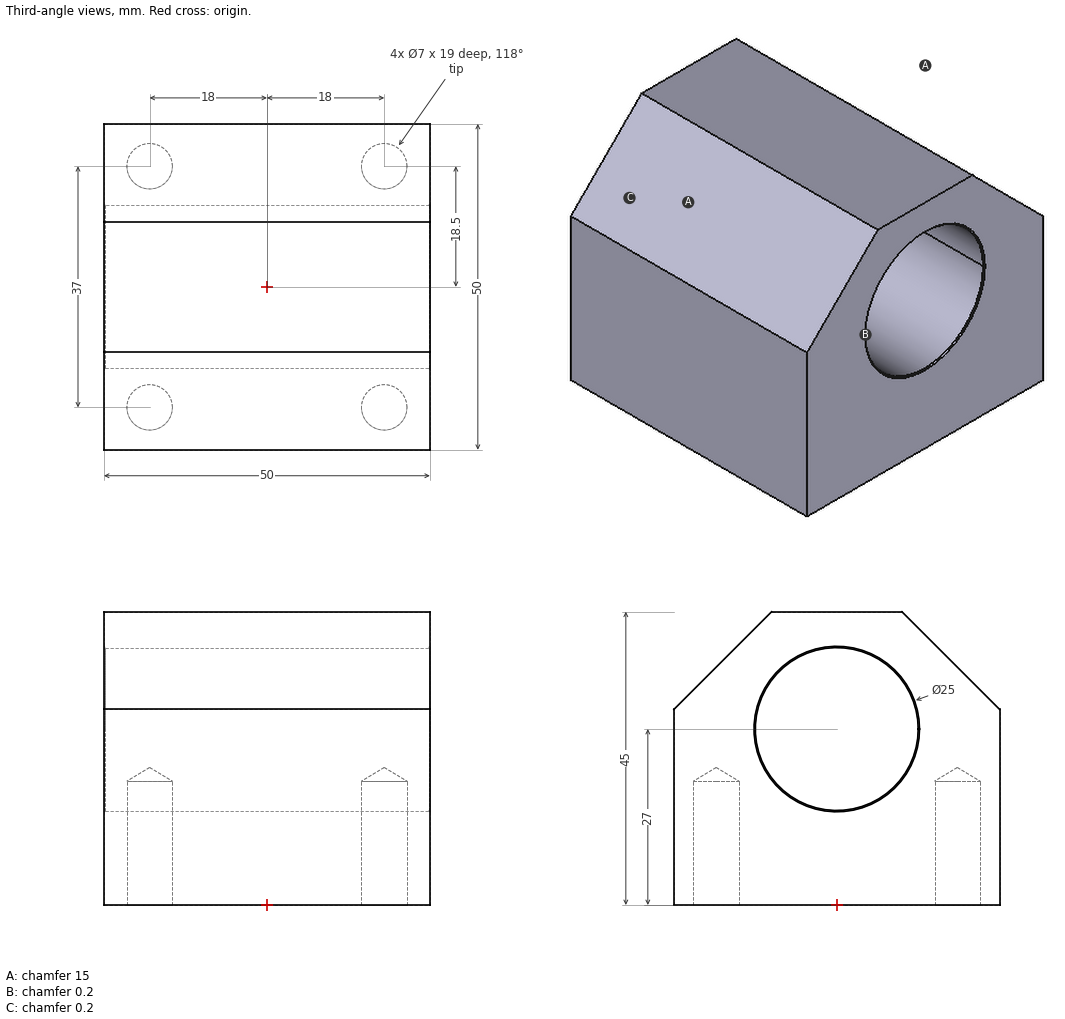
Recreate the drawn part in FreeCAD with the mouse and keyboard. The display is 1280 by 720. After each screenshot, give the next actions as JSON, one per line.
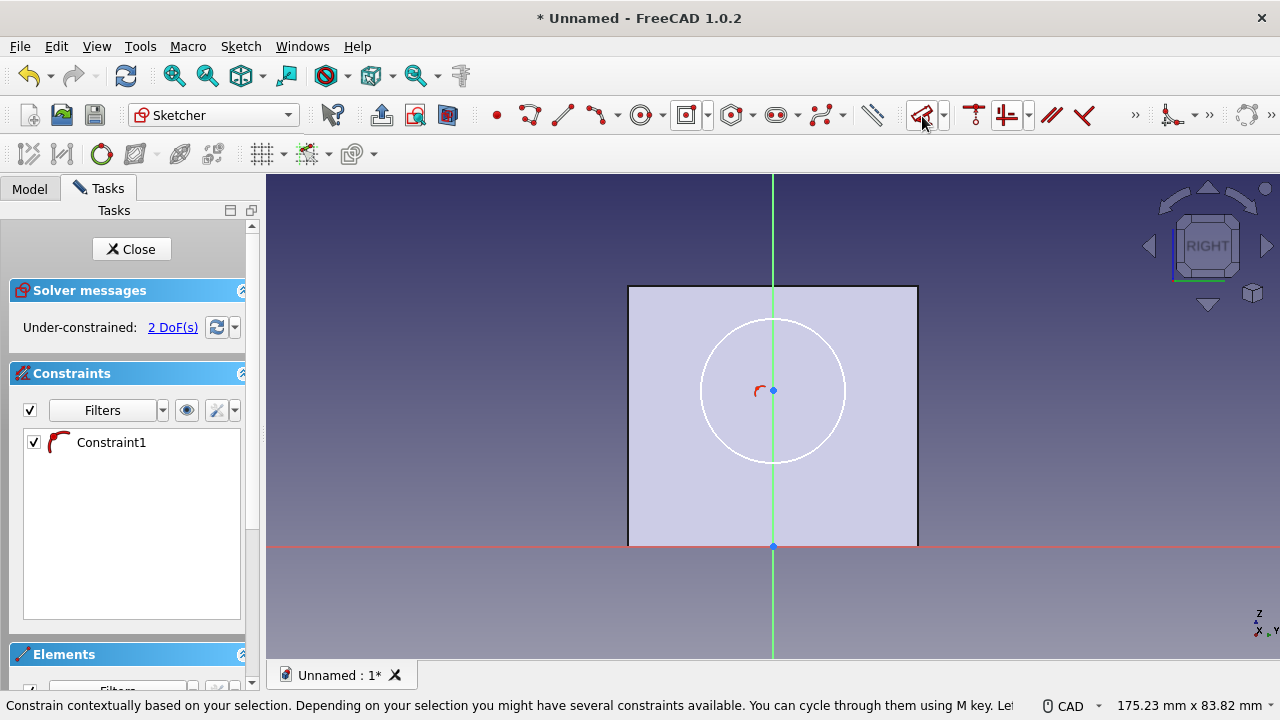
{"action": "left_click", "coordinate": [824, 340]}
{"action": "left_click", "coordinate": [847, 317]}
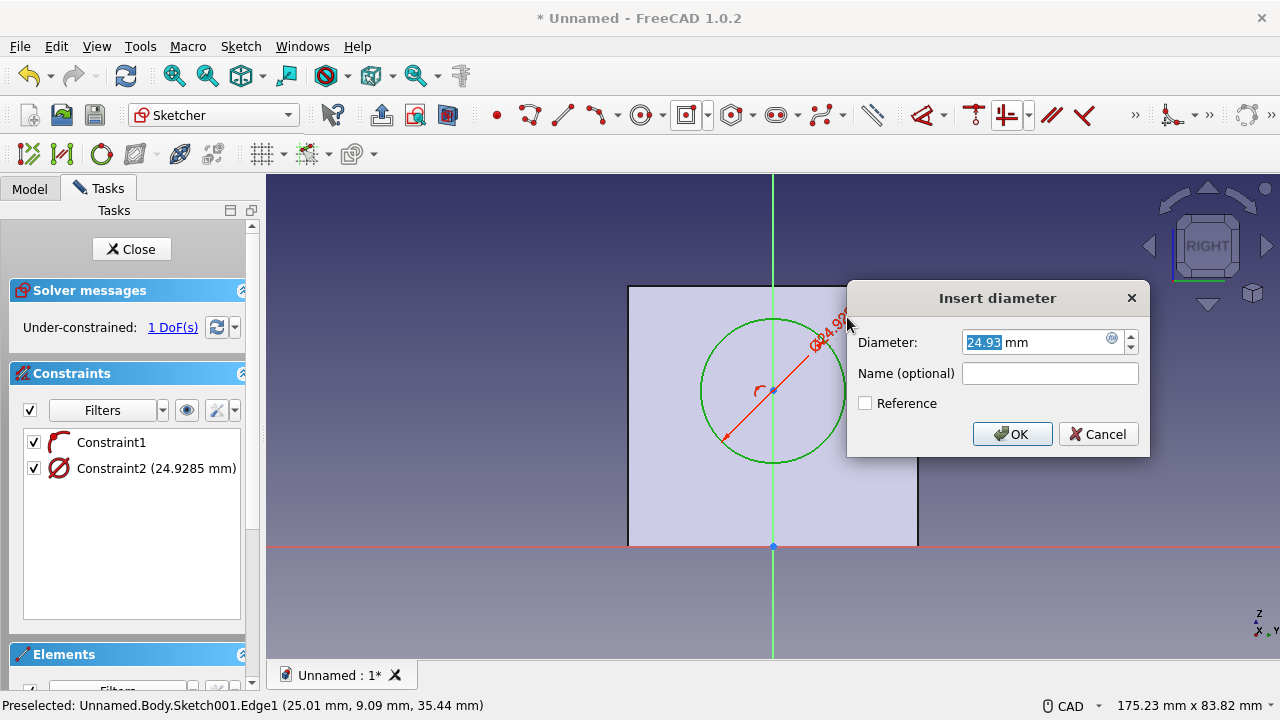
{"action": "type", "text": "25"}
{"action": "key", "text": "Return"}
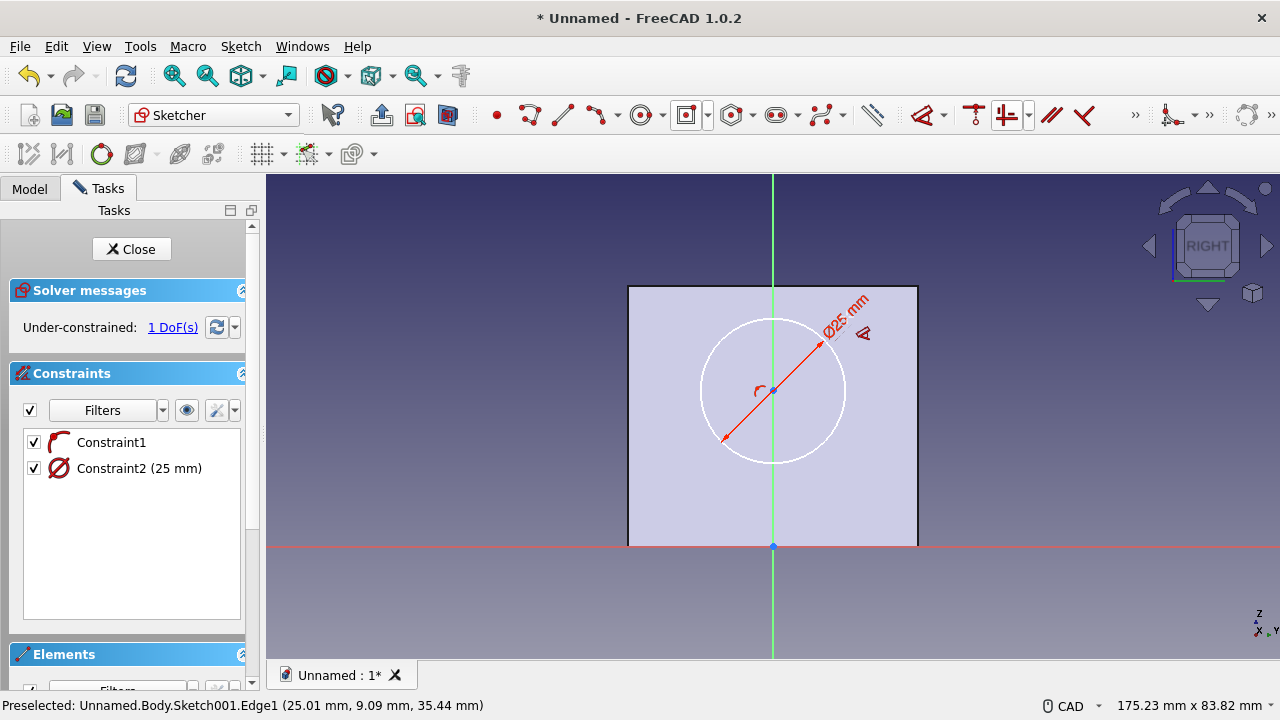
{"action": "left_click", "coordinate": [773, 391]}
{"action": "left_click", "coordinate": [807, 433]}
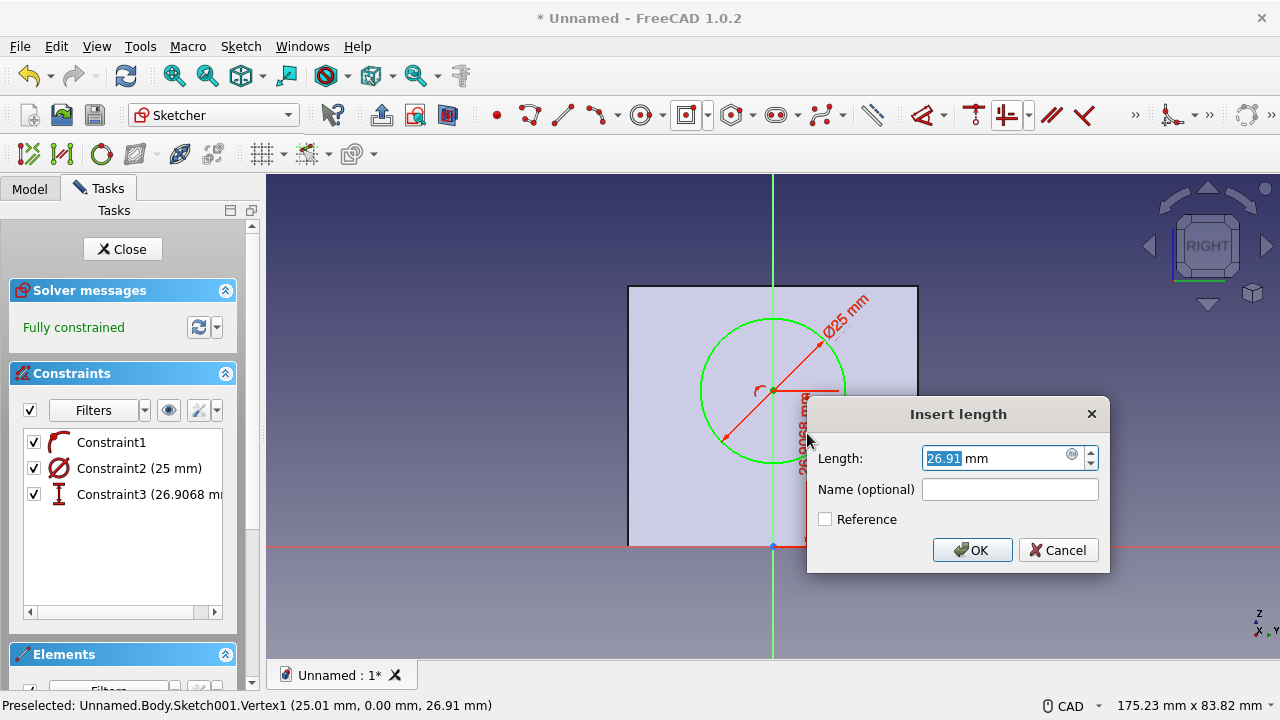
{"action": "type", "text": "27"}
{"action": "key", "text": "Return"}
{"action": "key", "text": "Escape"}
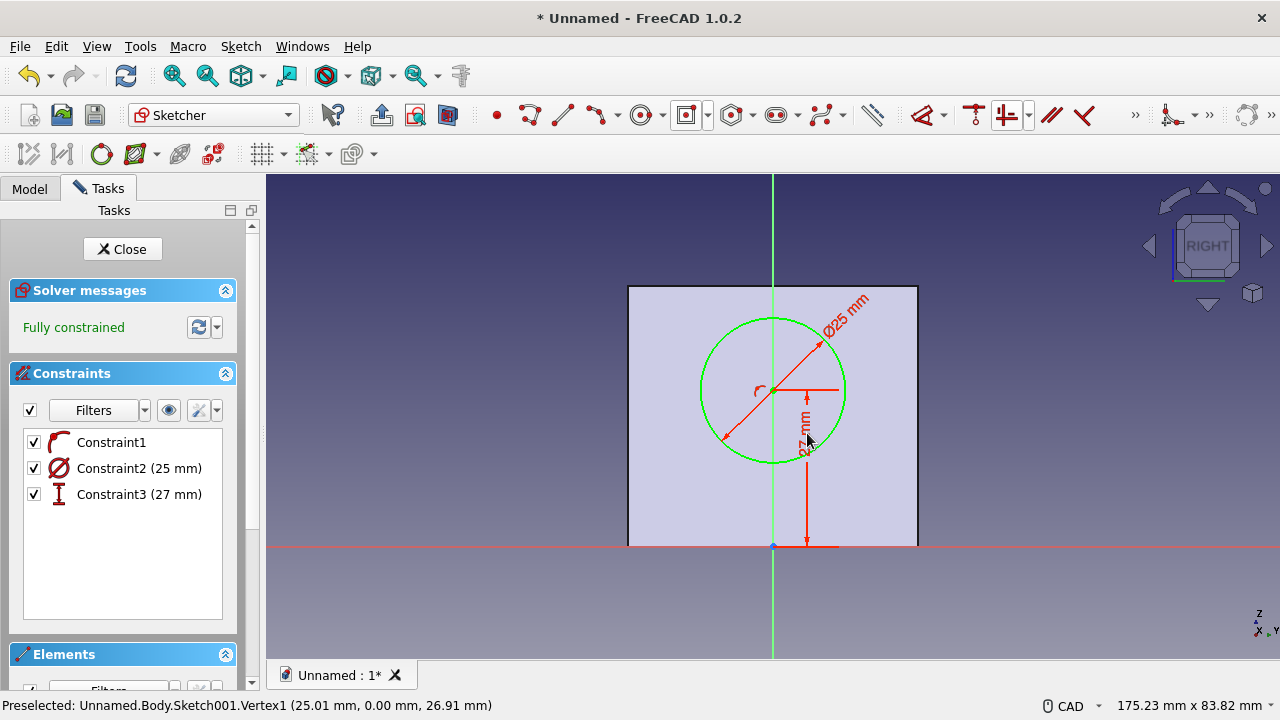
{"action": "left_click", "coordinate": [123, 249]}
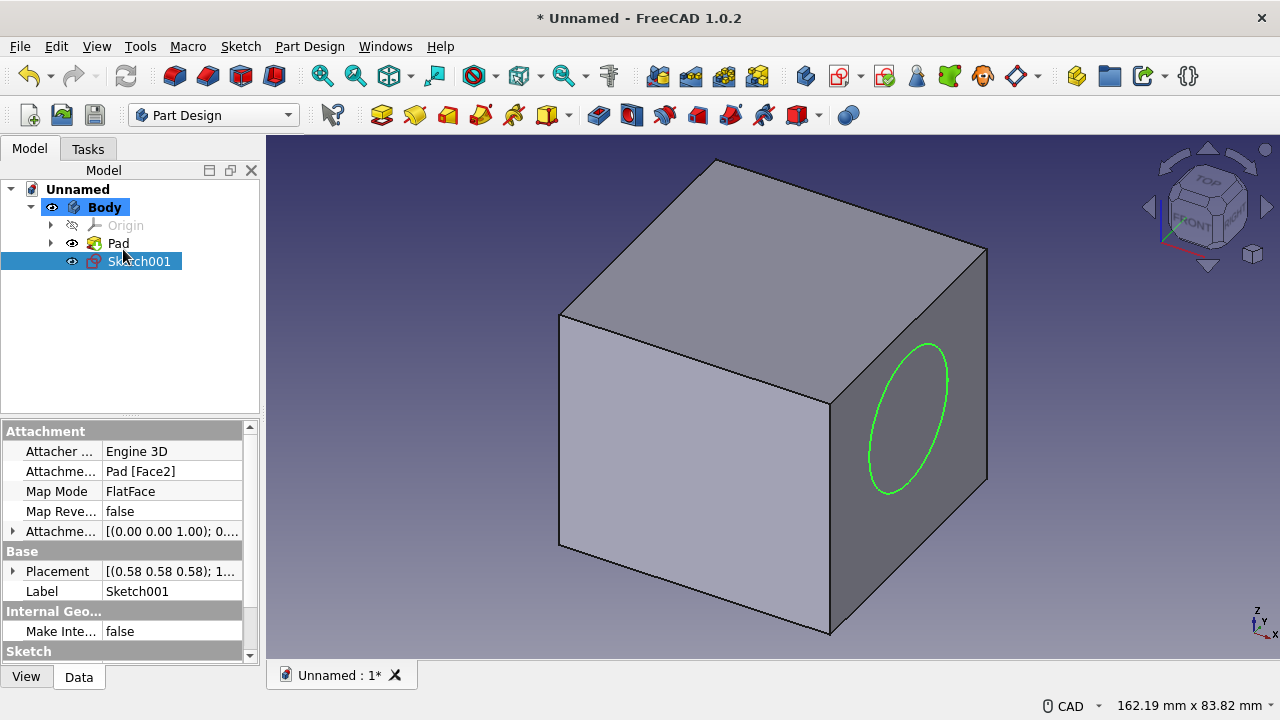
{"action": "left_click", "coordinate": [599, 116]}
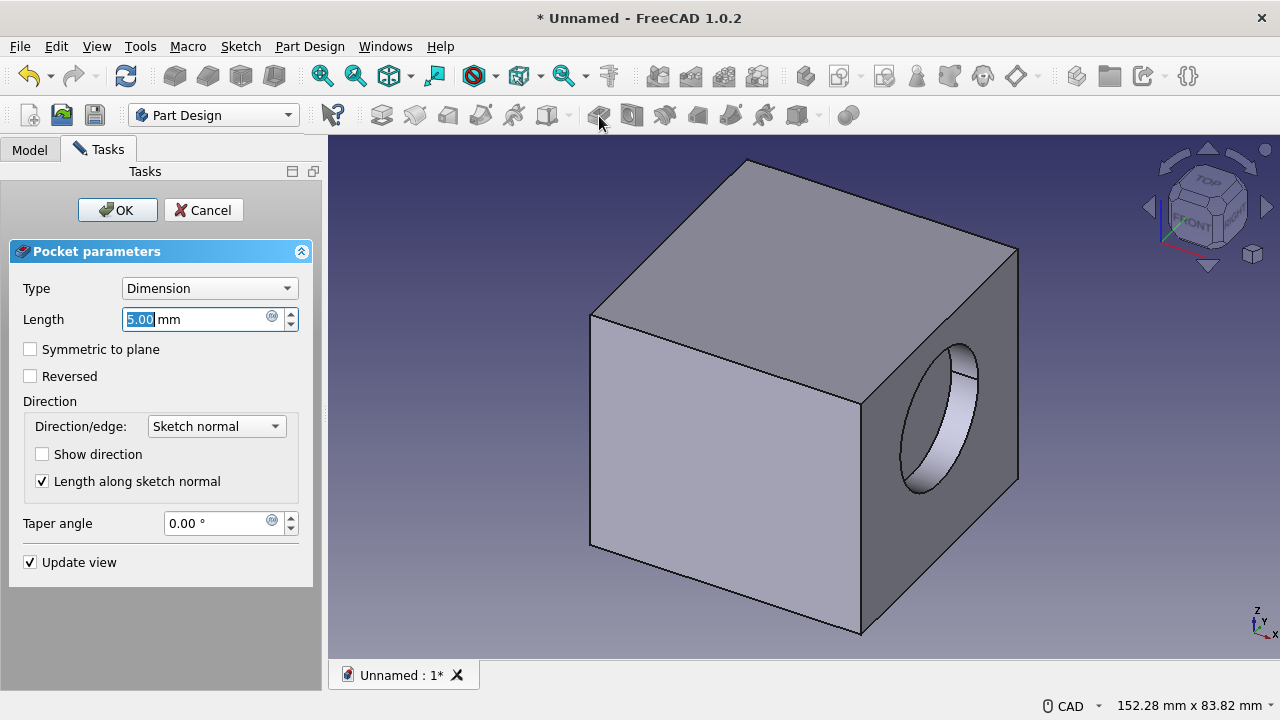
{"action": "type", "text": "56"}
{"action": "key", "text": "Tab"}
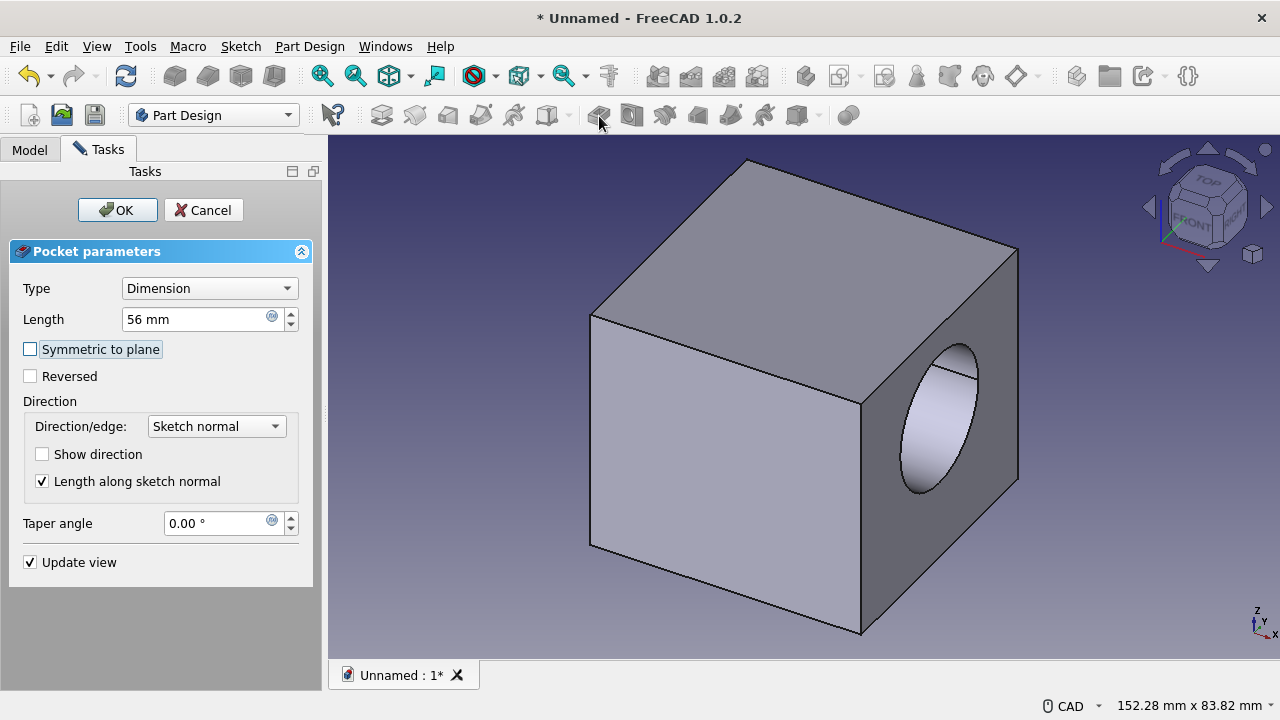
{"action": "left_click", "coordinate": [118, 210]}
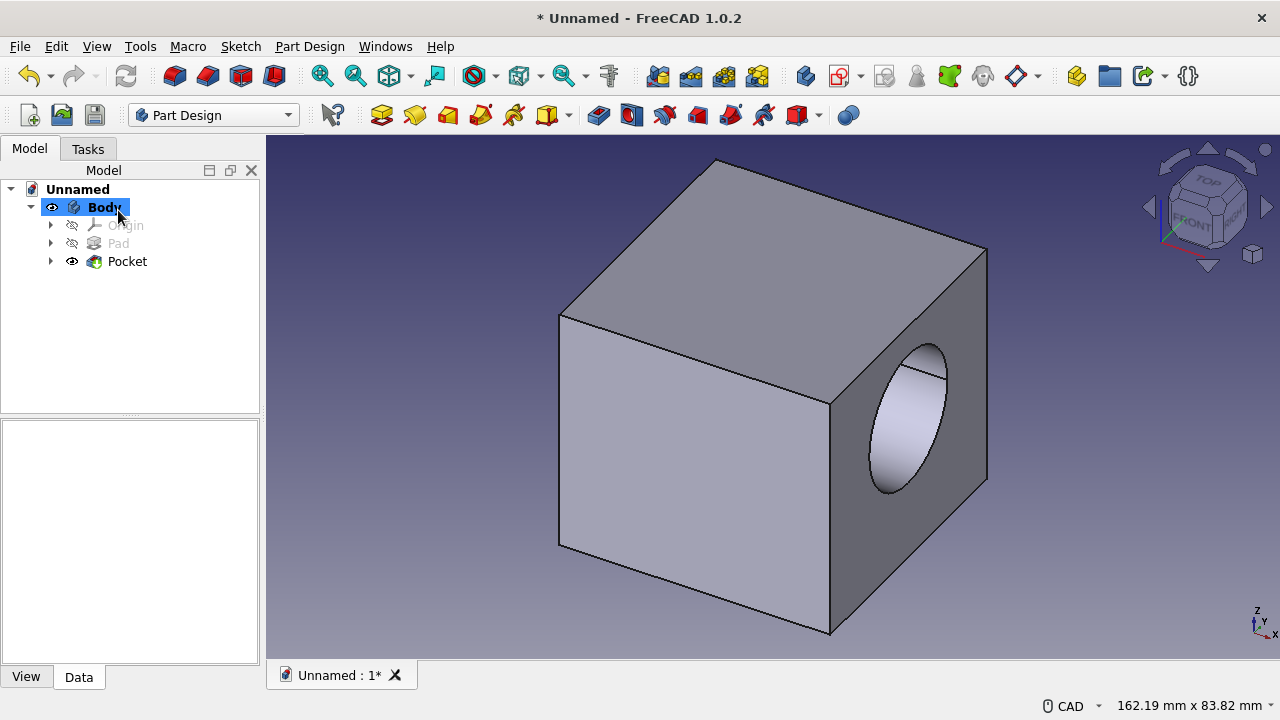
{"action": "left_click", "coordinate": [695, 358]}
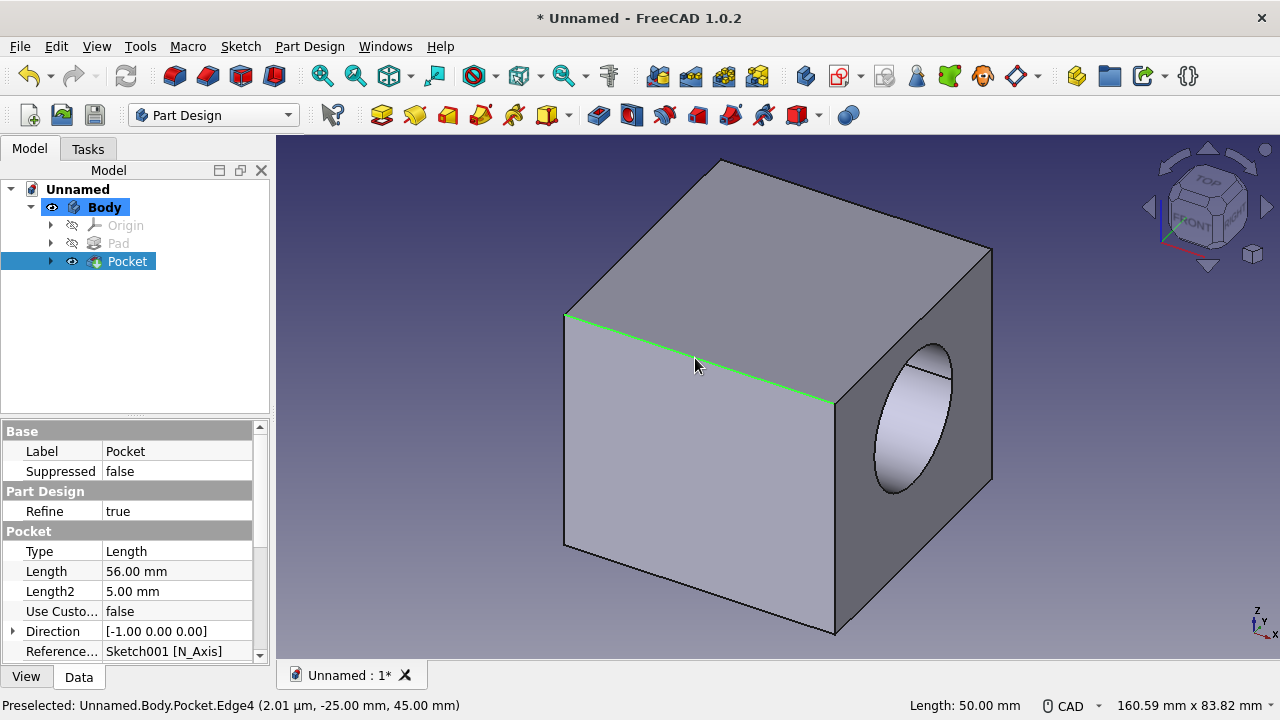
{"action": "key", "text": "0"}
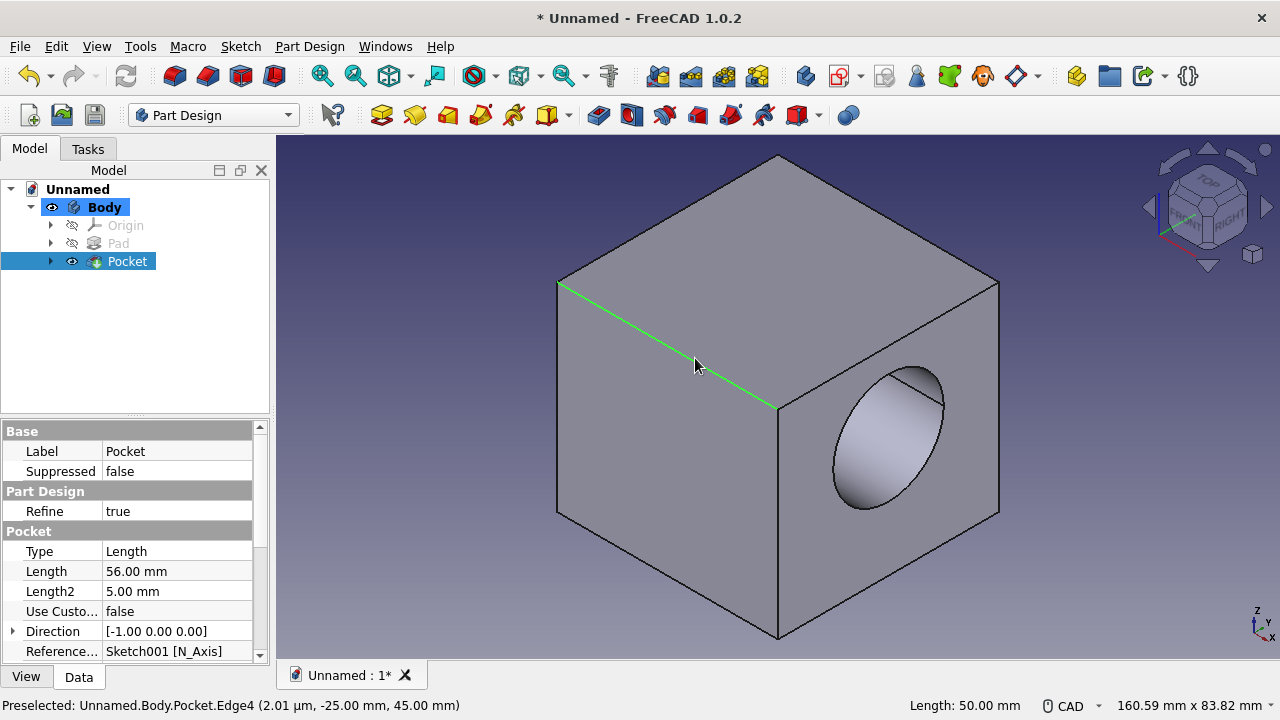
{"action": "key", "text": "2"}